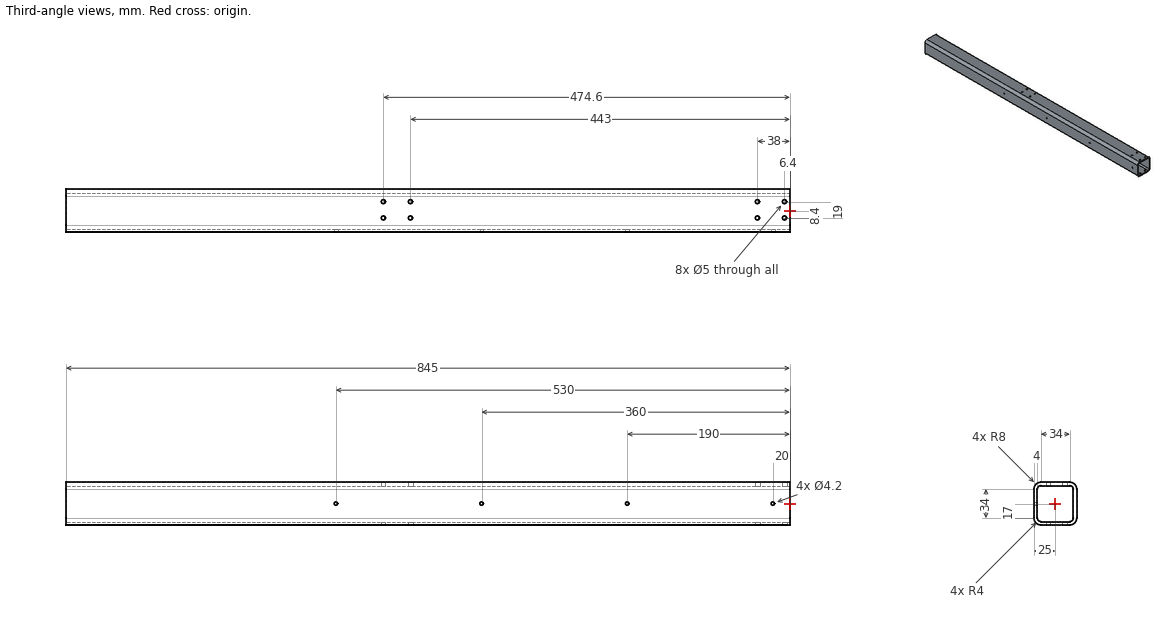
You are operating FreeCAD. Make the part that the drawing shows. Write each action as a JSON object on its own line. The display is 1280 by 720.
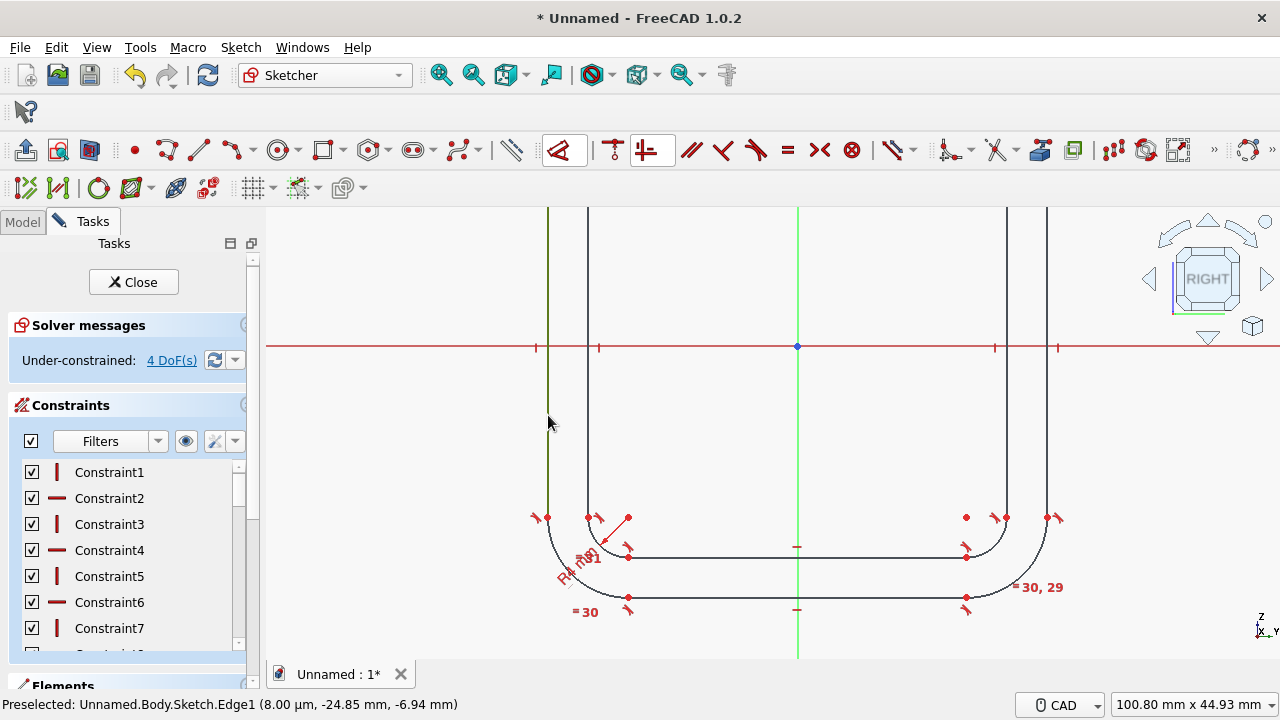
{"action": "key", "text": "i"}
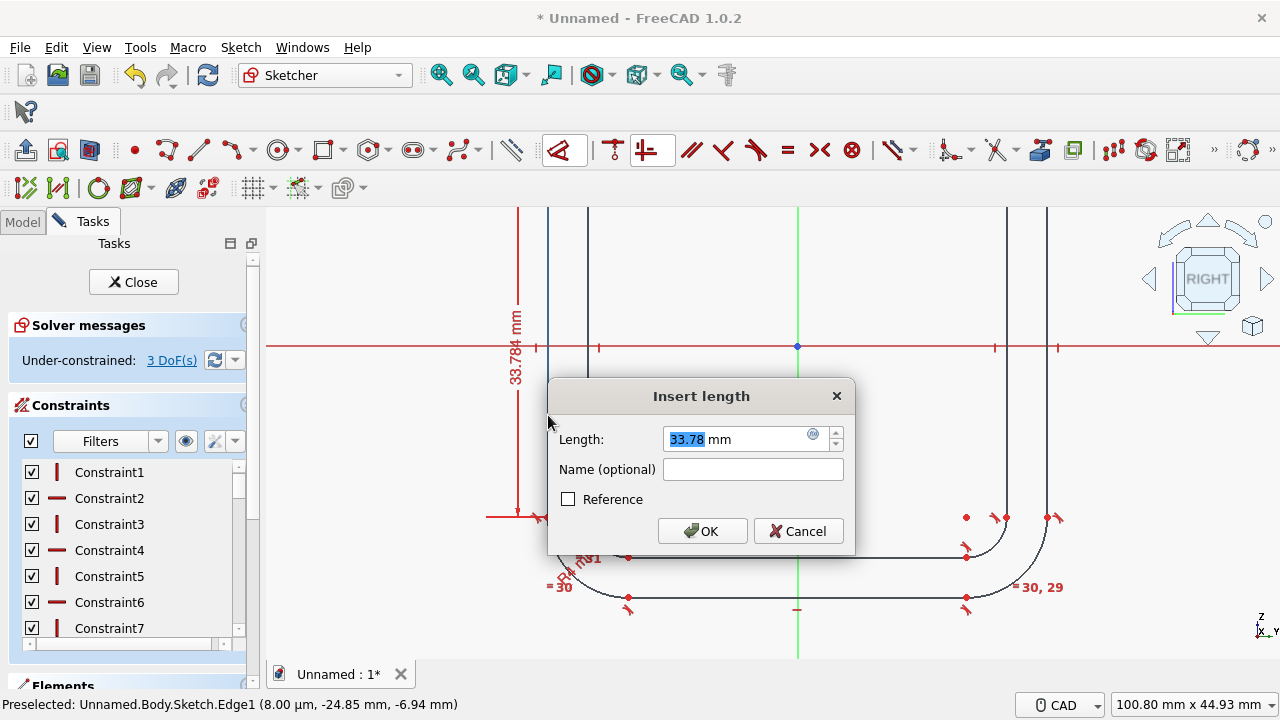
{"action": "type", "text": "34"}
{"action": "key", "text": "Return"}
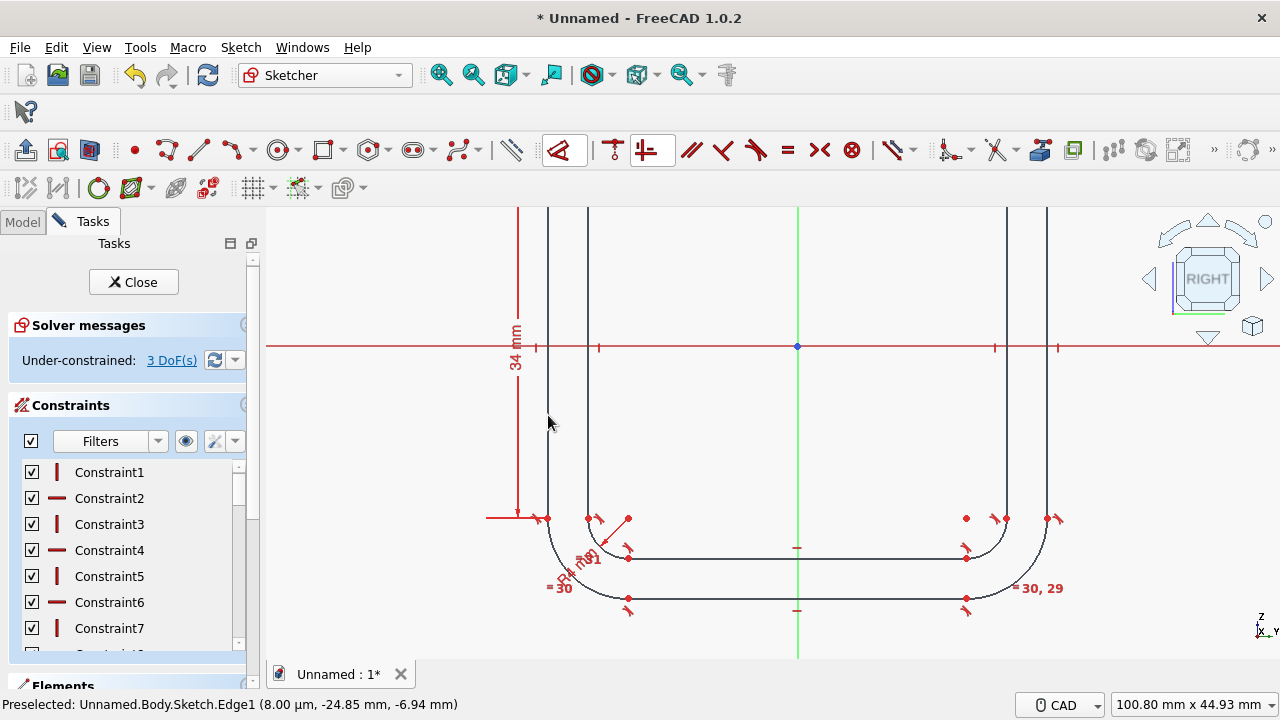
{"action": "scroll", "coordinate": [591, 539], "scroll_direction": "down", "scroll_amount": 3}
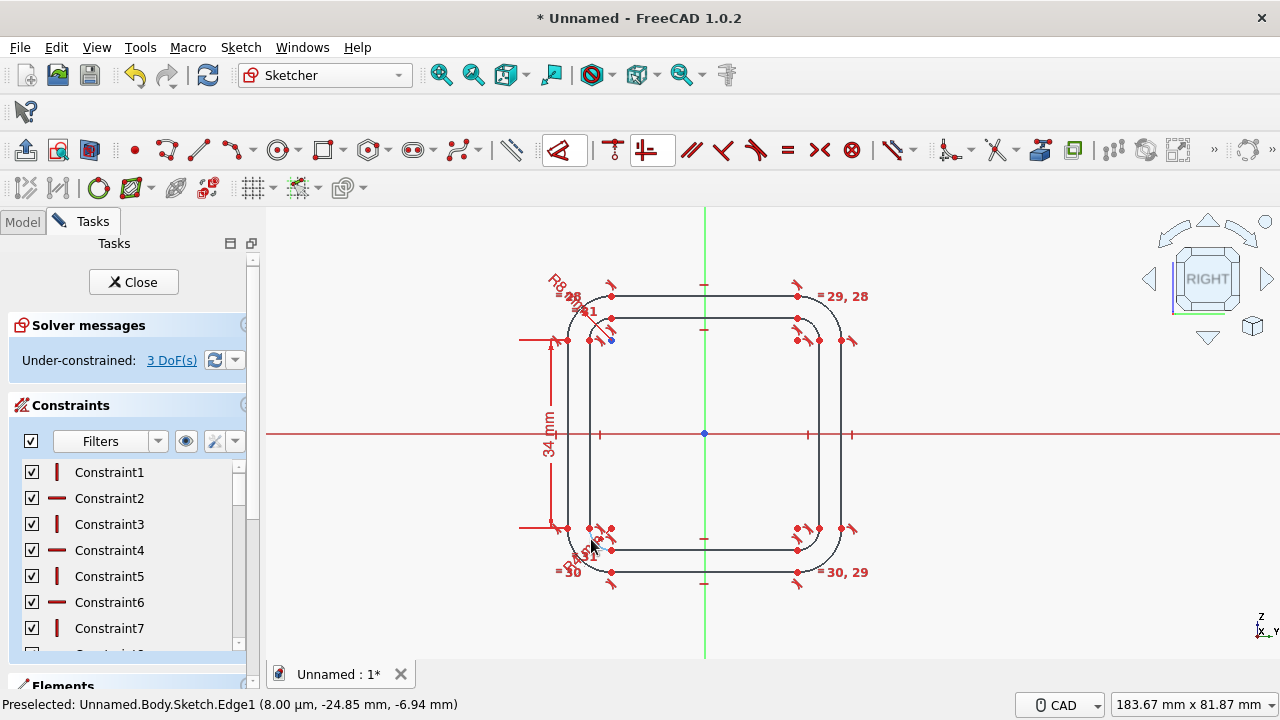
{"action": "left_click", "coordinate": [667, 296]}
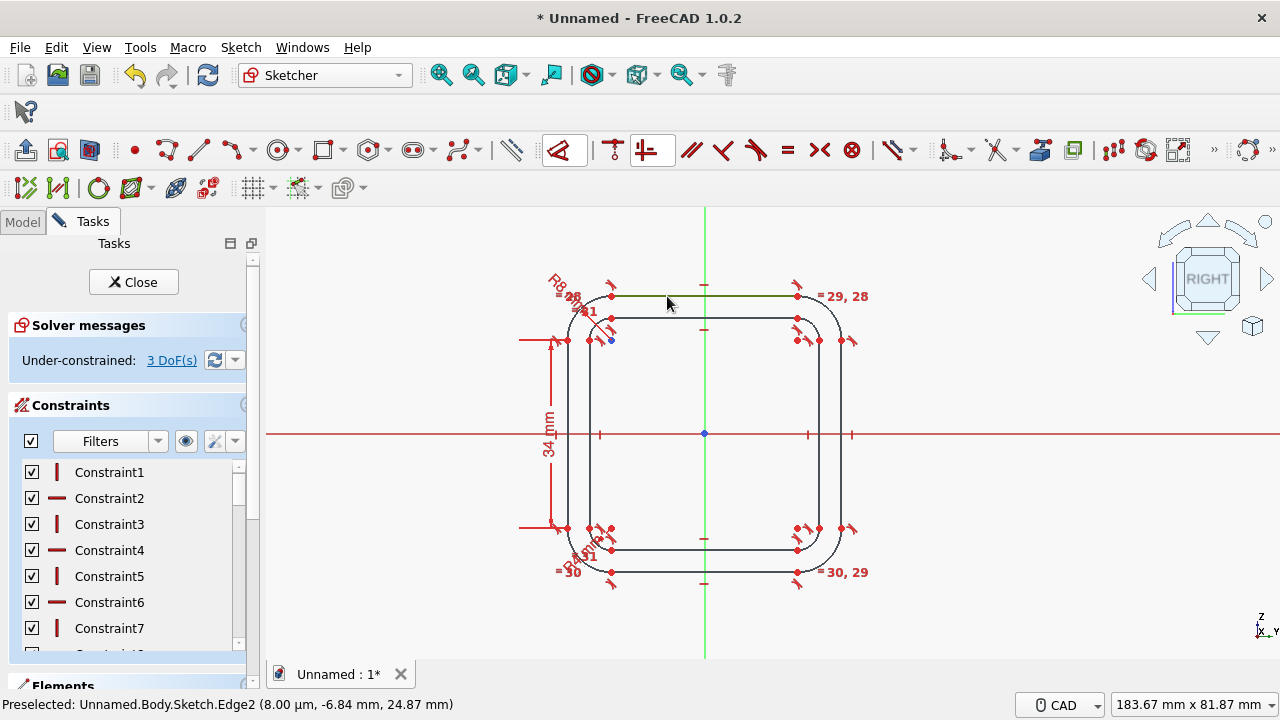
{"action": "key", "text": "l"}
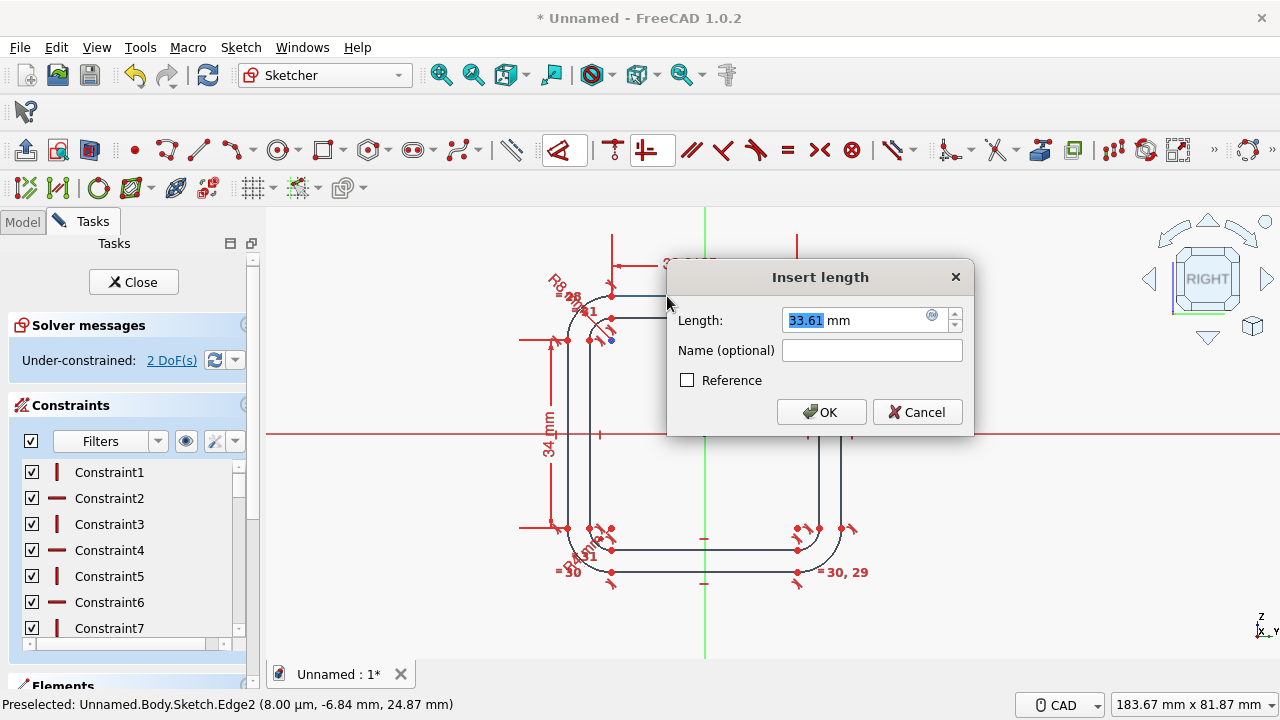
{"action": "type", "text": "34"}
{"action": "key", "text": "Return"}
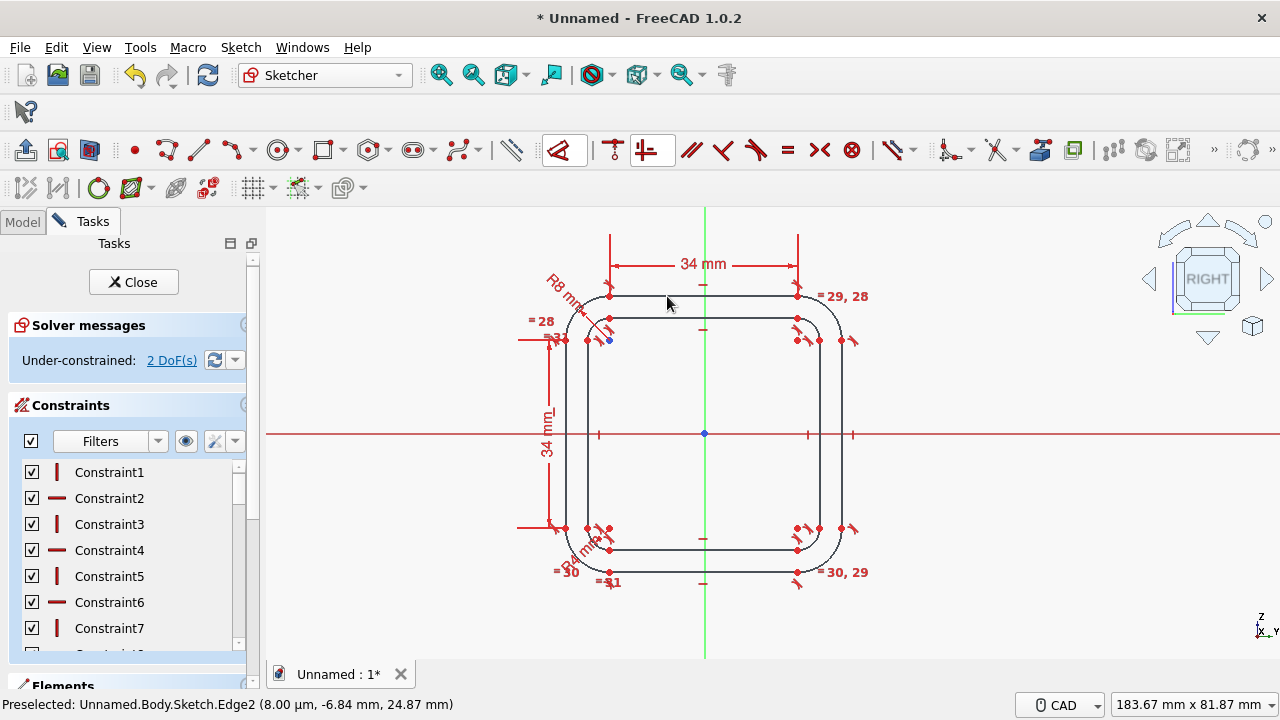
{"action": "left_click", "coordinate": [566, 528]}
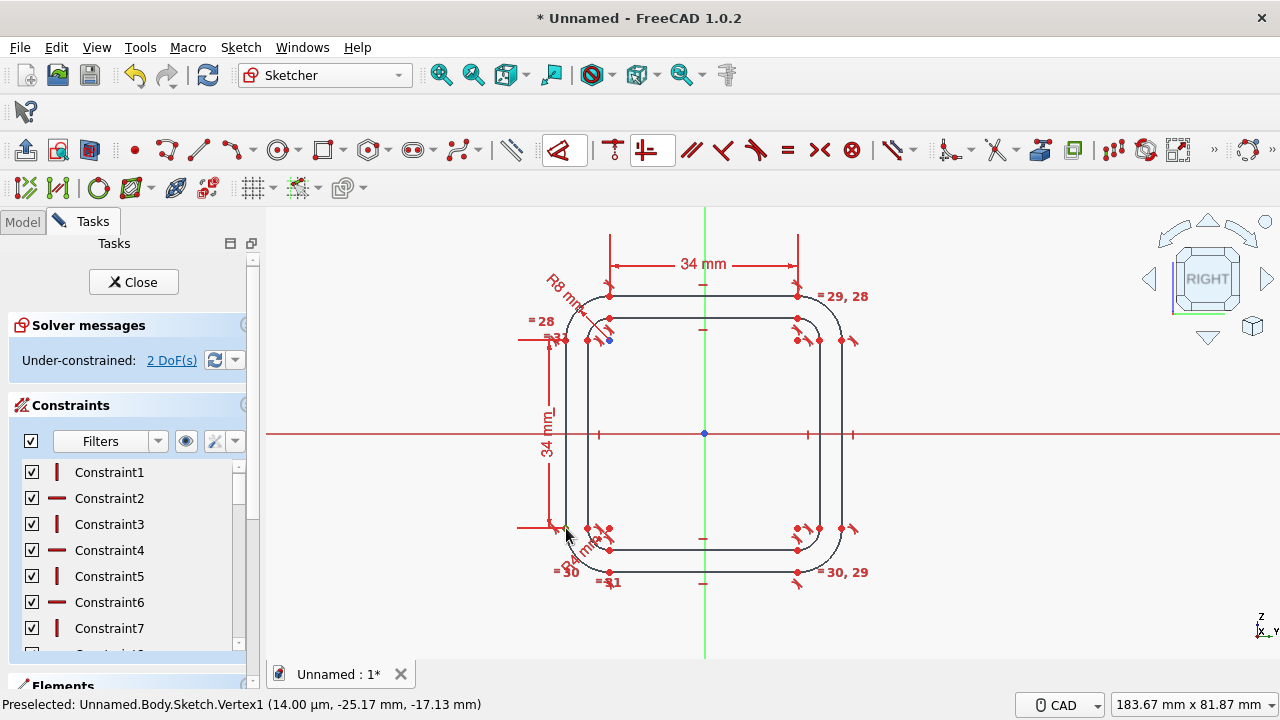
{"action": "key", "text": "l"}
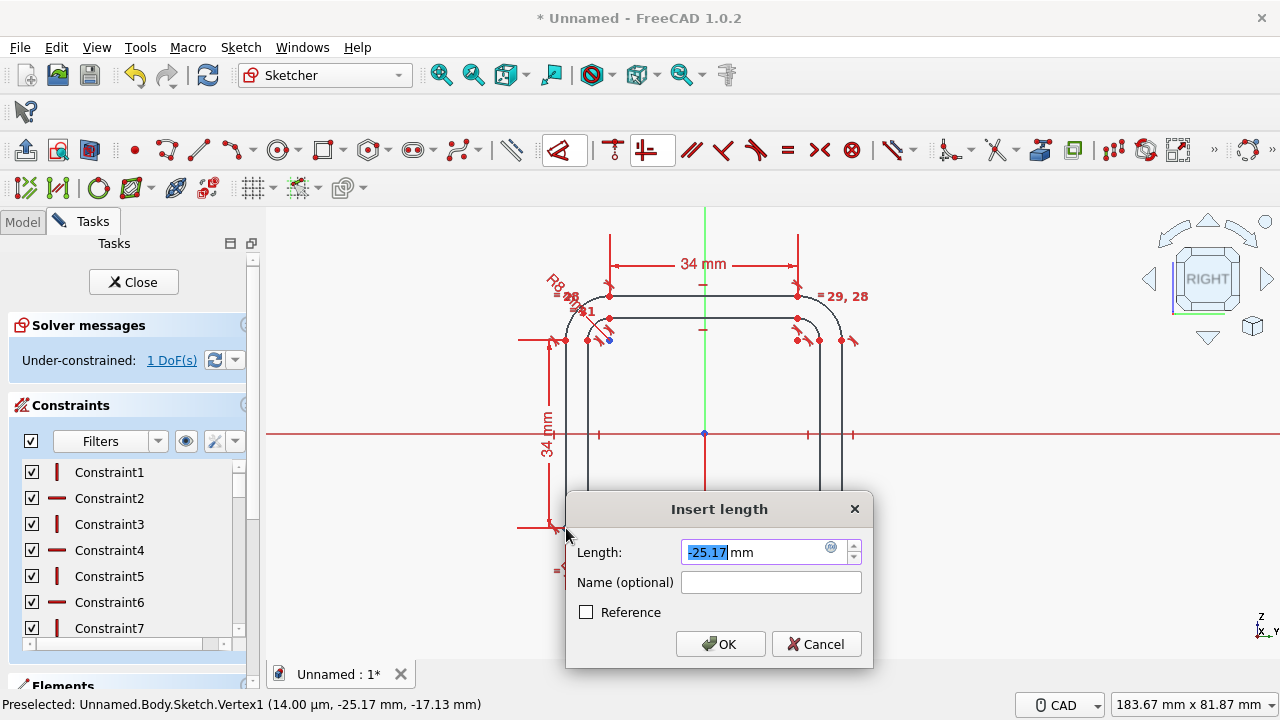
{"action": "type", "text": "-25"}
{"action": "key", "text": "Return"}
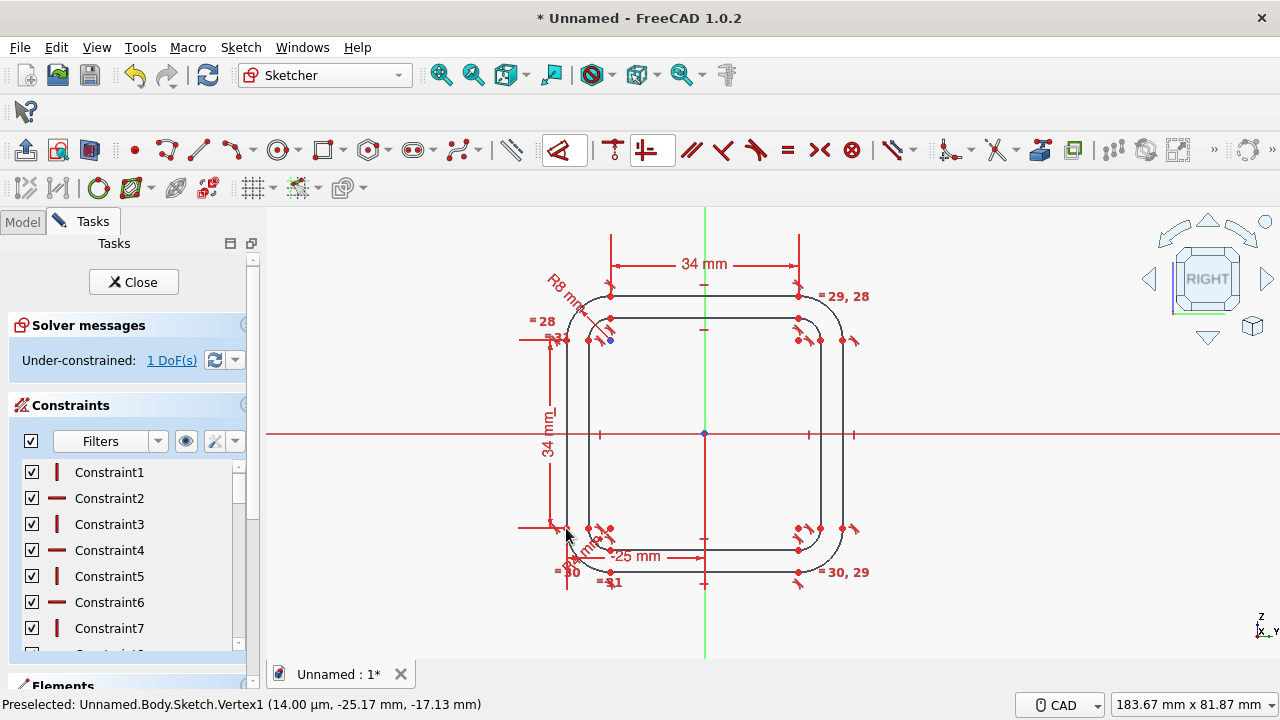
{"action": "left_click", "coordinate": [567, 528]}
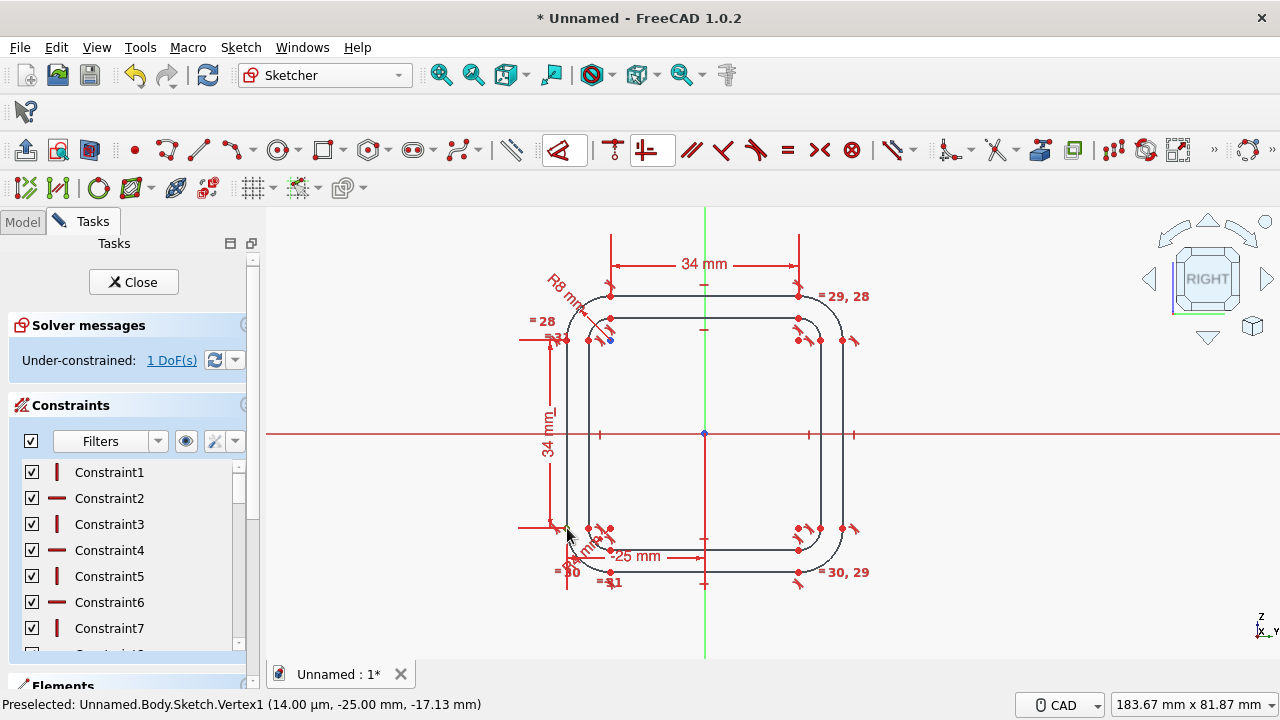
{"action": "left_click", "coordinate": [582, 150]}